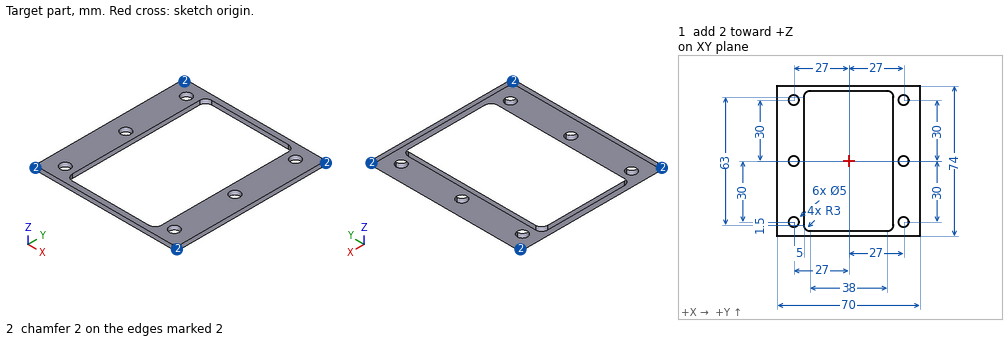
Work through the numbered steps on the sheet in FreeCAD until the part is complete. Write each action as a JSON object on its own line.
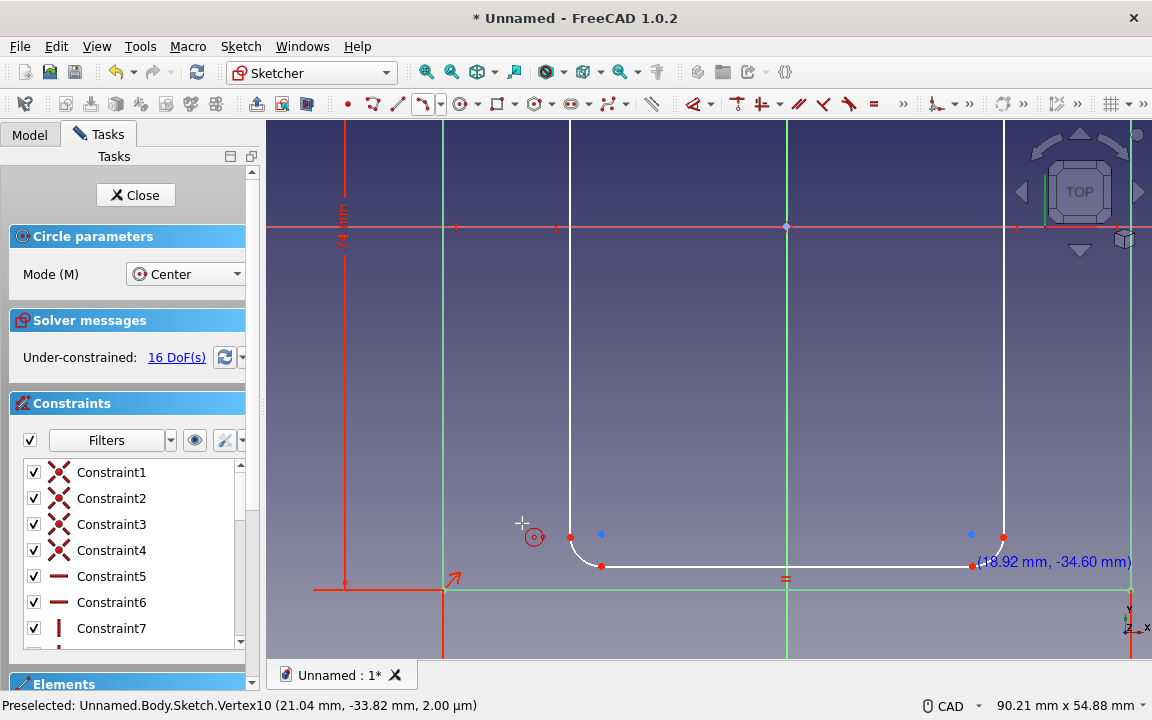
{"action": "left_click", "coordinate": [522, 521]}
{"action": "mouse_move", "coordinate": [539, 504]}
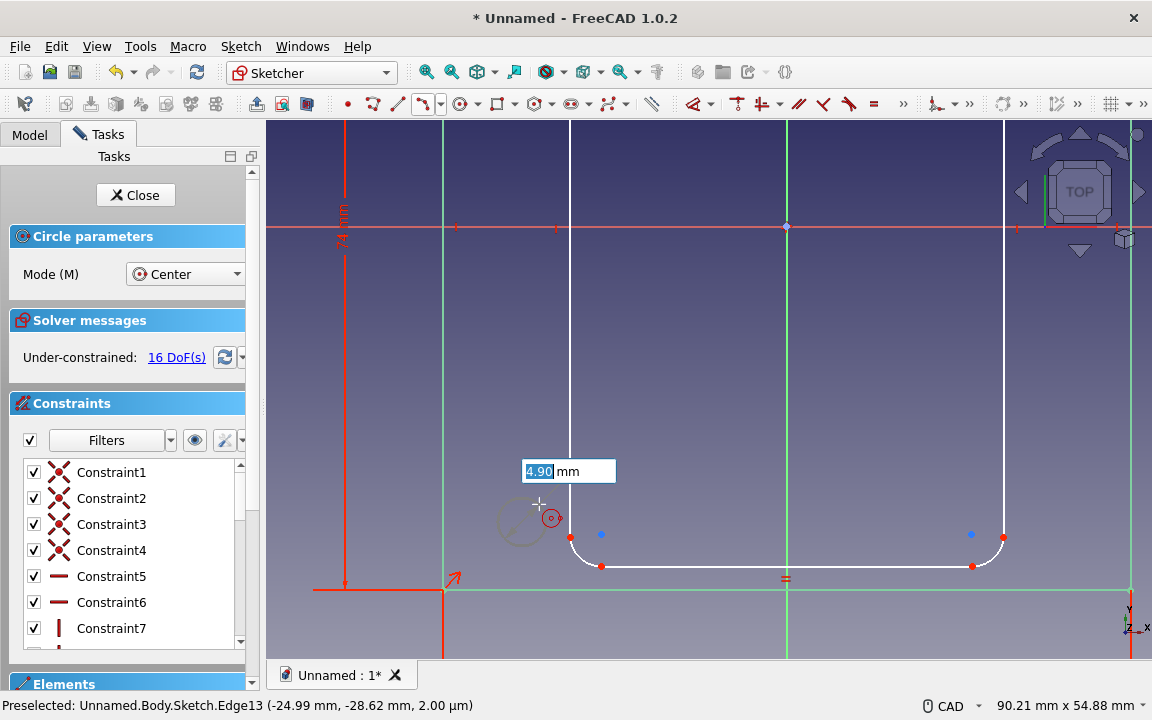
{"action": "type", "text": "5"}
{"action": "key", "text": "Return"}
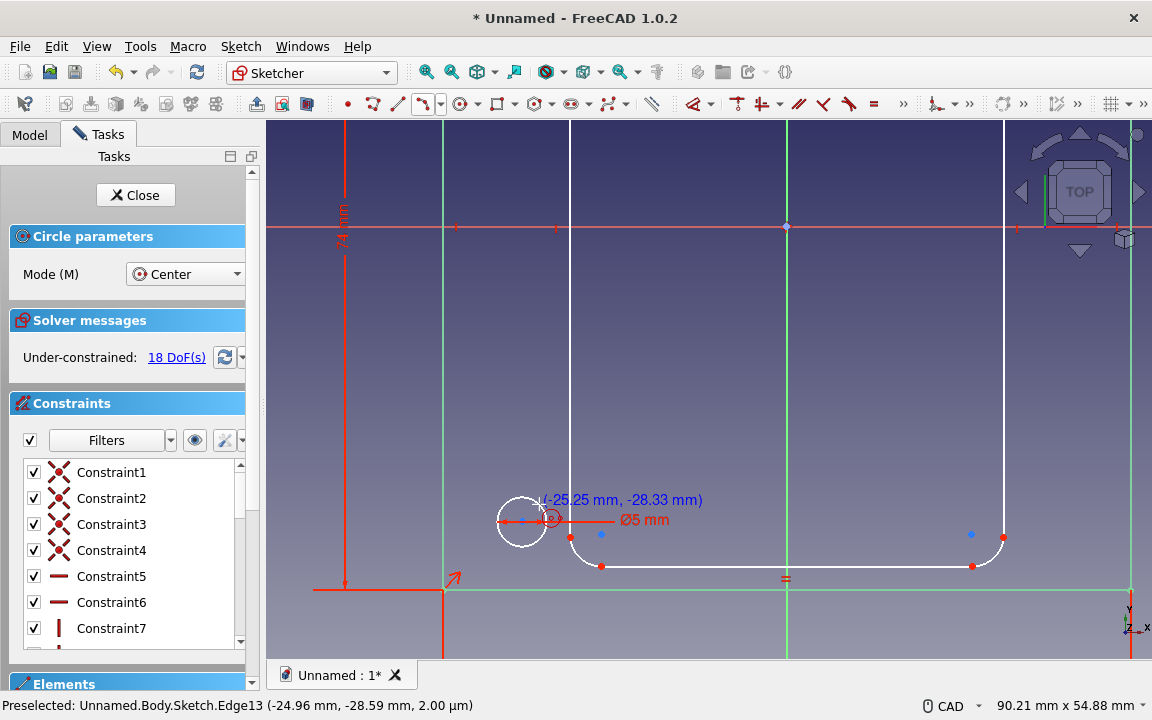
{"action": "scroll", "coordinate": [521, 522], "scroll_direction": "down", "scroll_amount": 4}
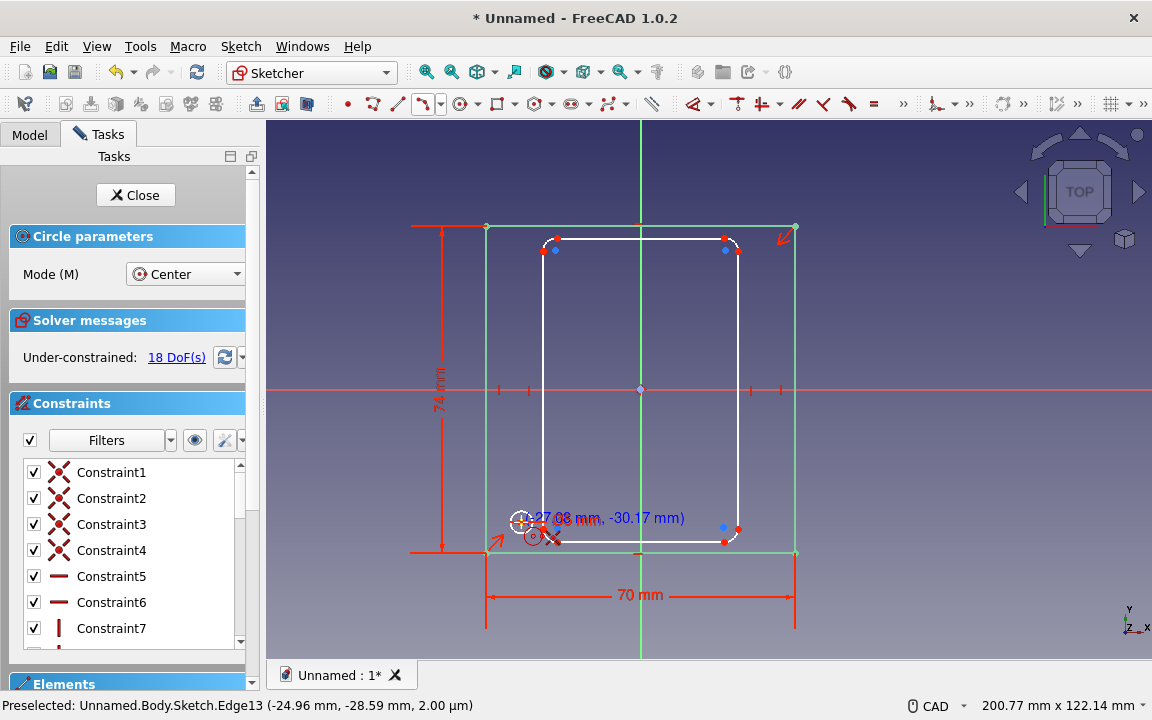
{"action": "scroll", "coordinate": [760, 522], "scroll_direction": "up", "scroll_amount": 4}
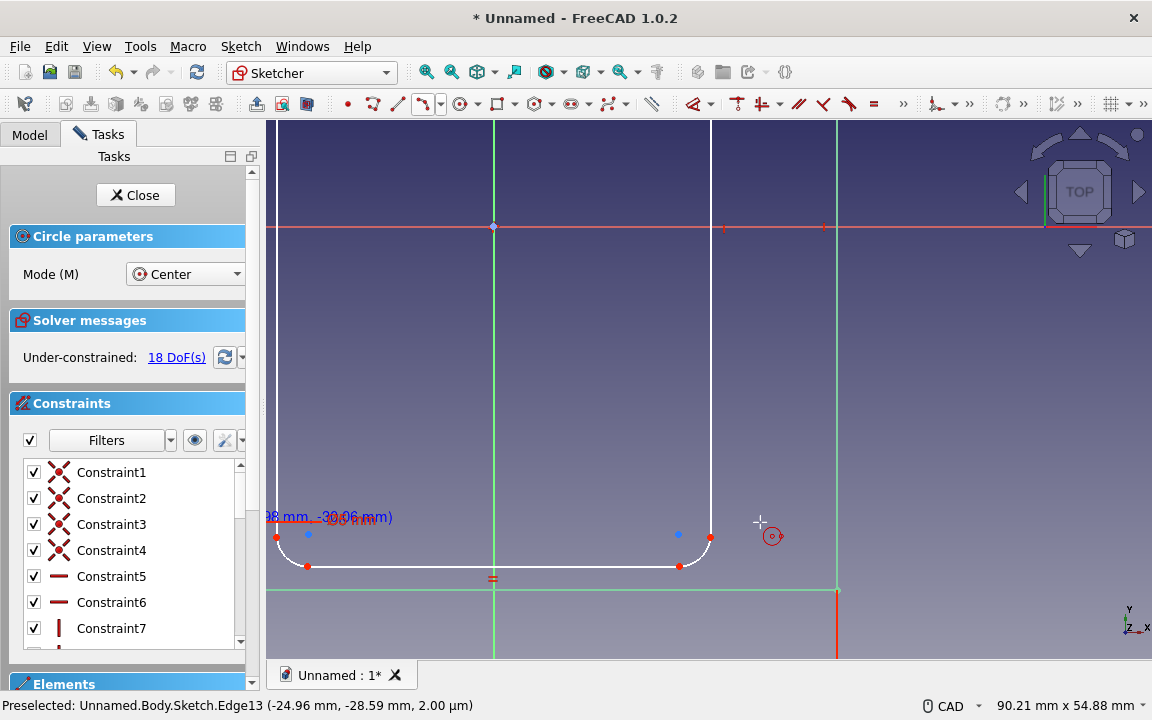
{"action": "left_click", "coordinate": [759, 521]}
{"action": "mouse_move", "coordinate": [776, 504]}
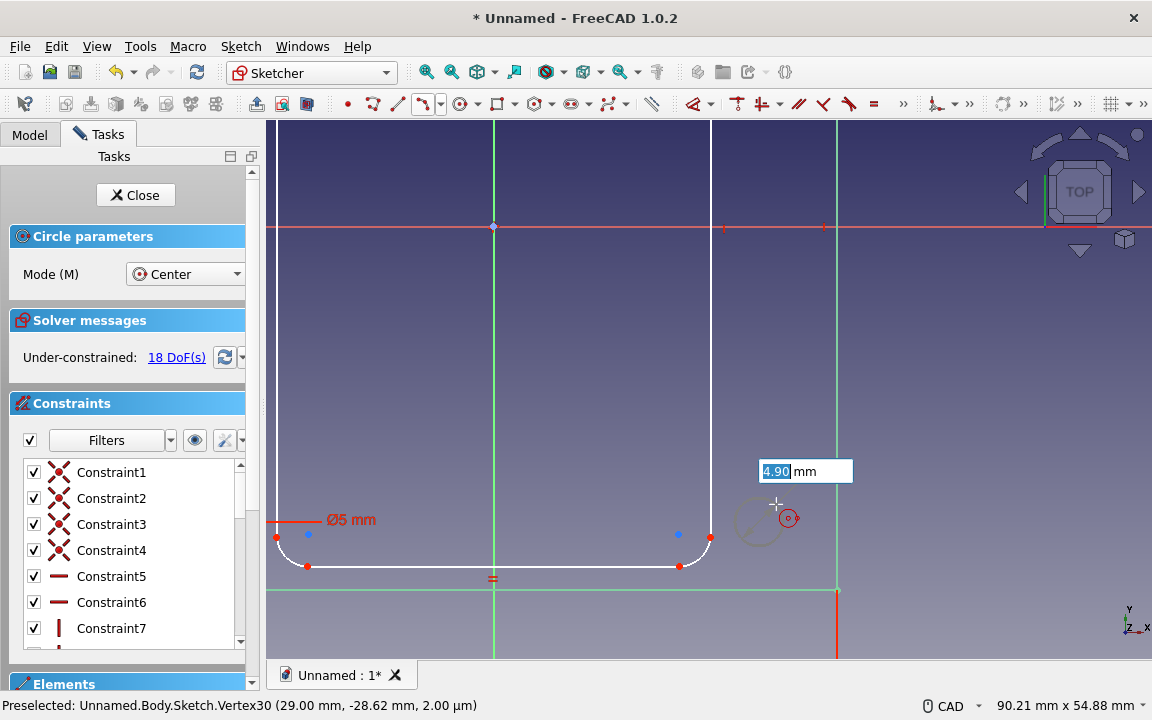
{"action": "type", "text": "5"}
{"action": "key", "text": "Return"}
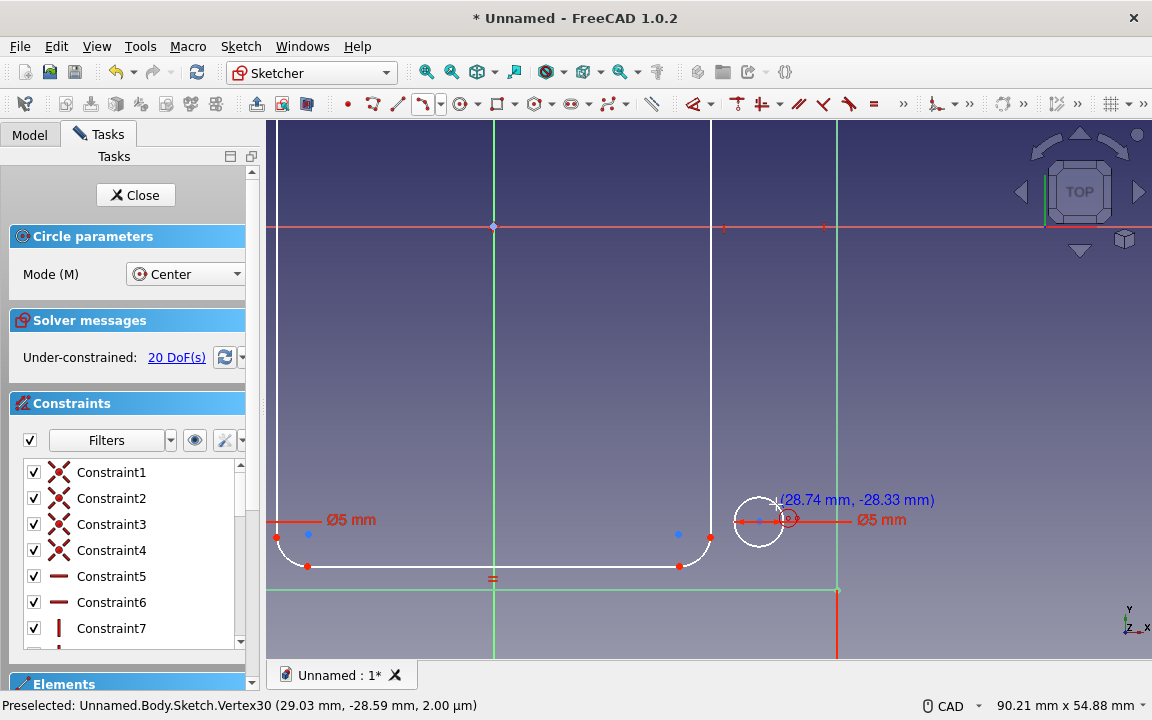
{"action": "scroll", "coordinate": [760, 522], "scroll_direction": "down", "scroll_amount": 4}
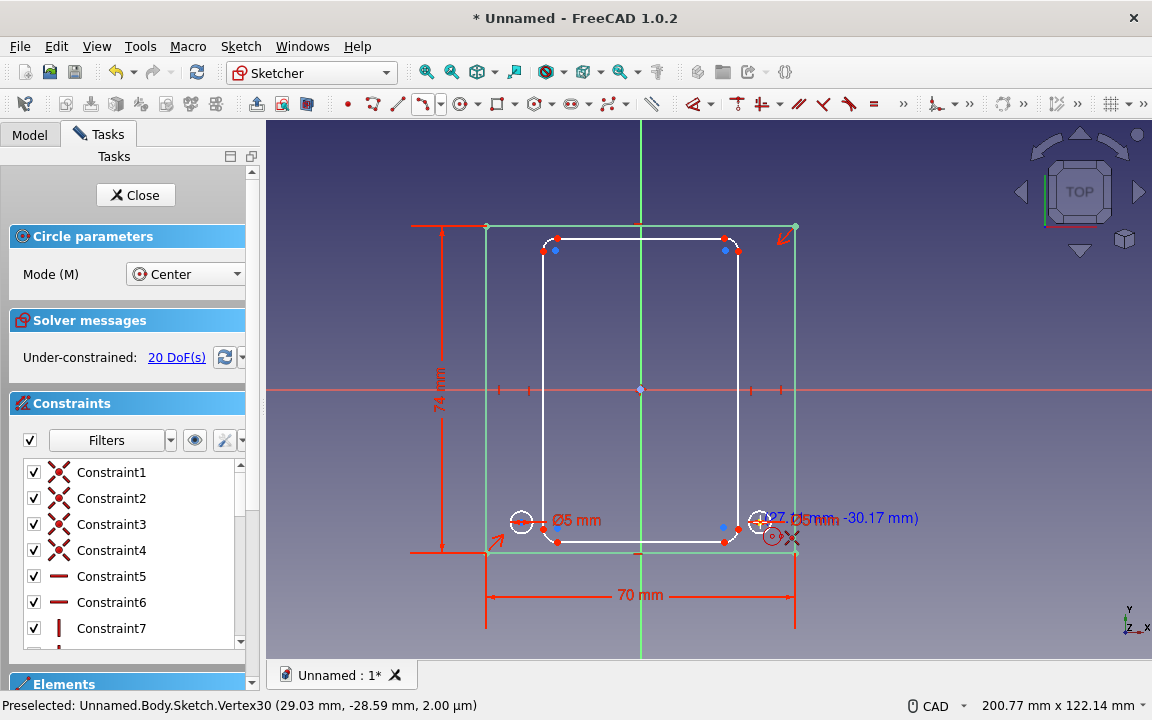
{"action": "scroll", "coordinate": [522, 390], "scroll_direction": "up", "scroll_amount": 4}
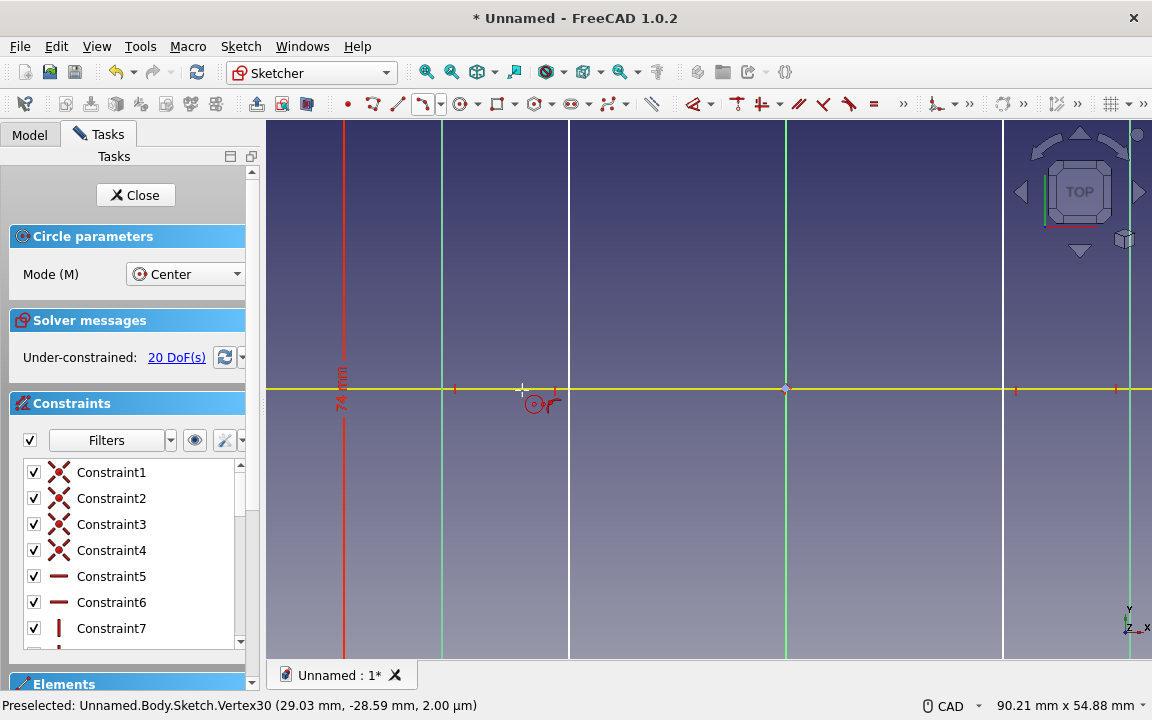
{"action": "left_click", "coordinate": [521, 389]}
{"action": "mouse_move", "coordinate": [538, 371]}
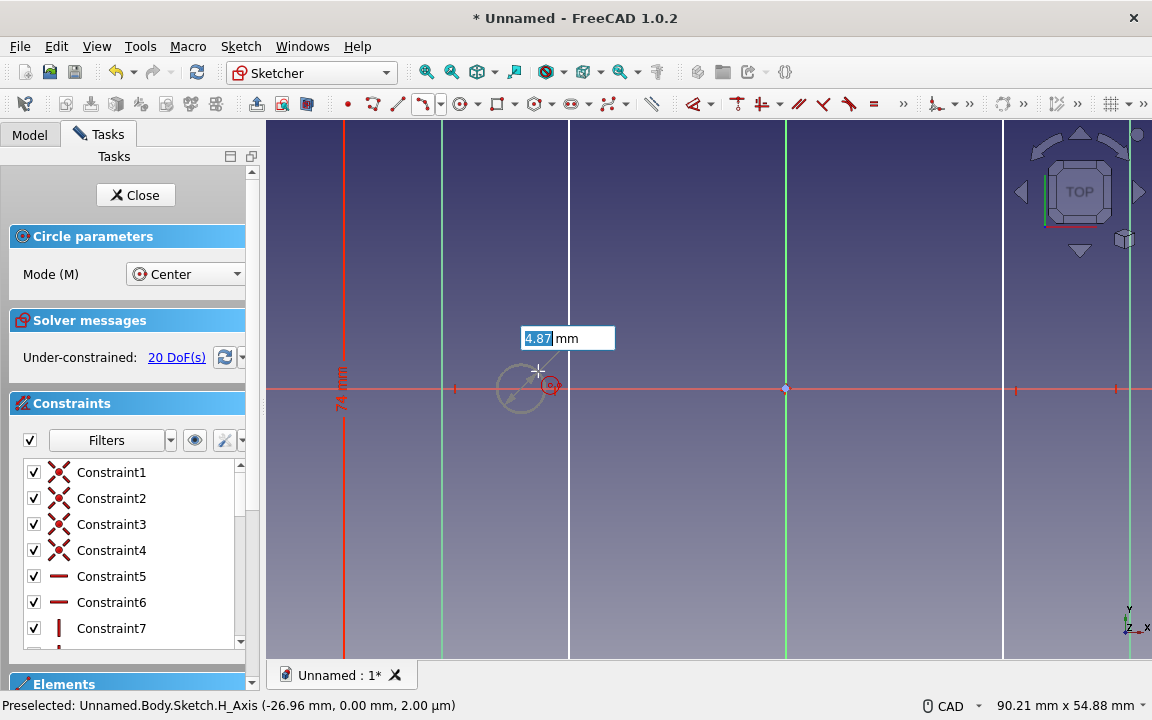
{"action": "type", "text": "5"}
{"action": "key", "text": "Return"}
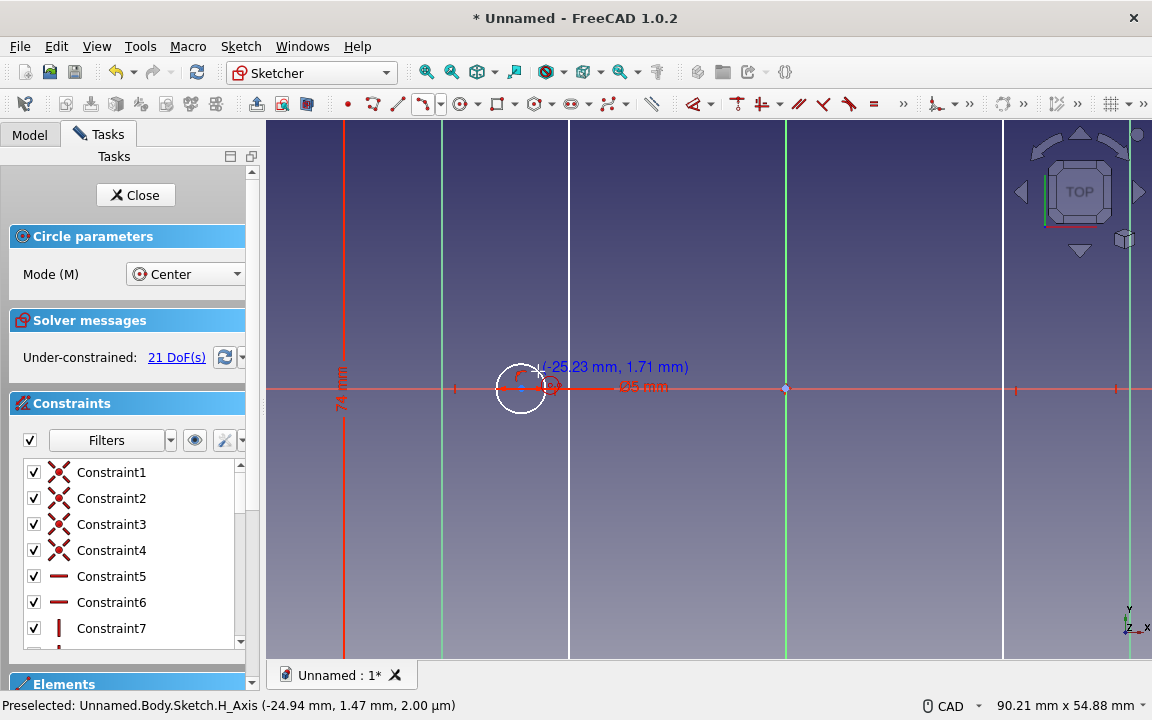
{"action": "scroll", "coordinate": [522, 390], "scroll_direction": "down", "scroll_amount": 4}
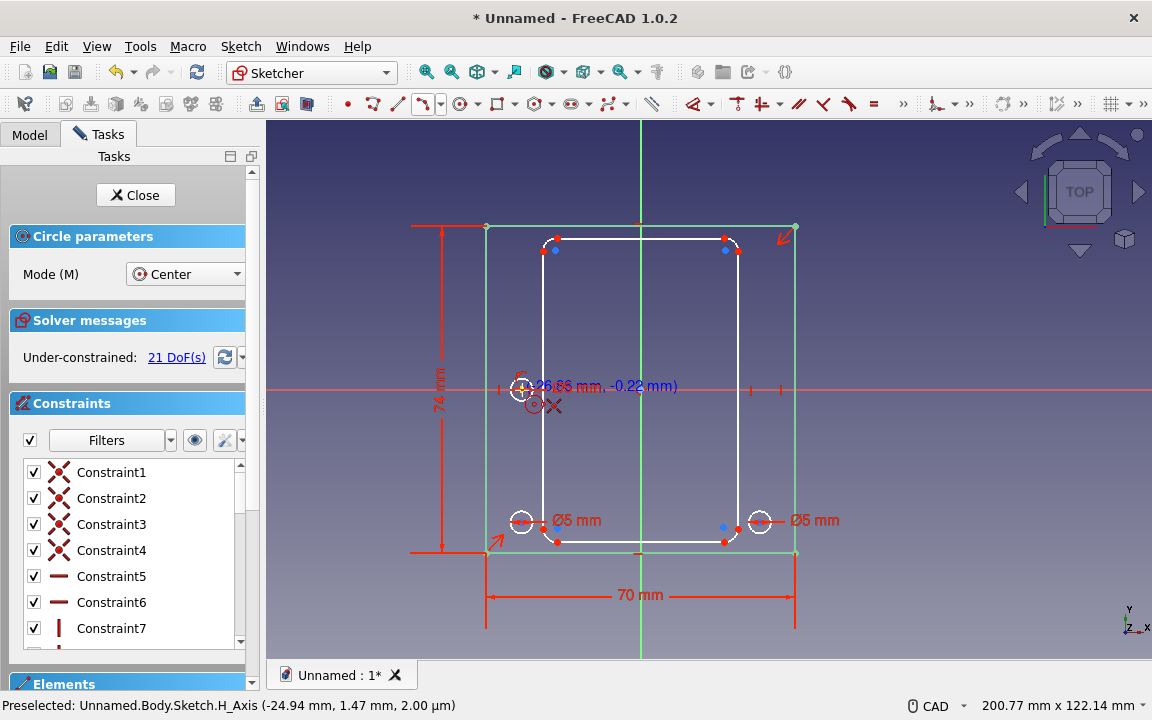
{"action": "scroll", "coordinate": [522, 257], "scroll_direction": "up", "scroll_amount": 4}